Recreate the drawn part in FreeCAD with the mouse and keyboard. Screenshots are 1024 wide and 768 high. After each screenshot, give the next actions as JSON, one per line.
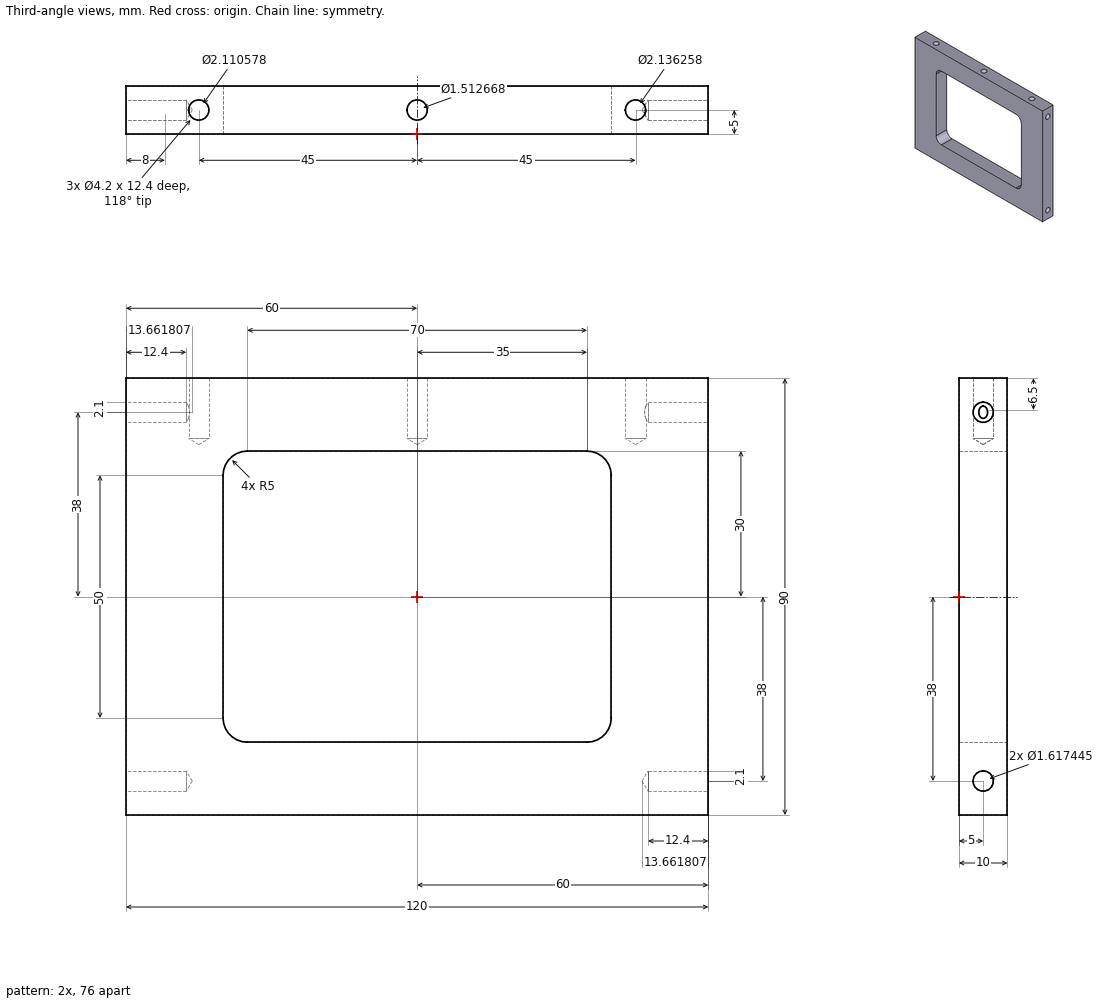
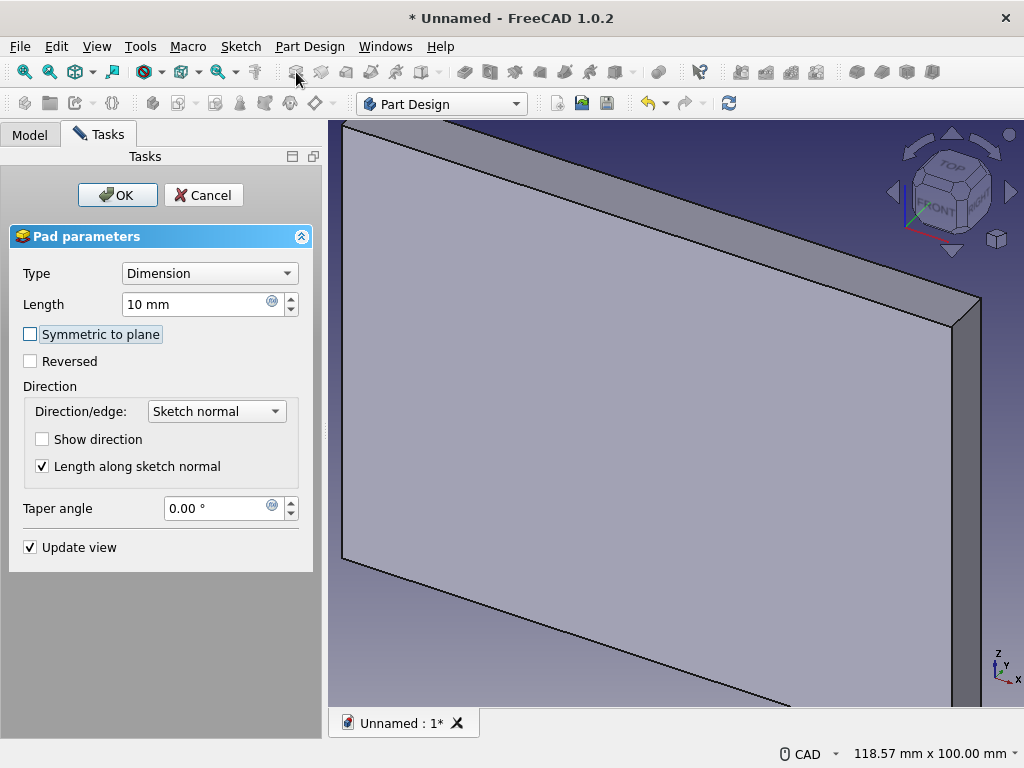
{"action": "left_click", "coordinate": [31, 361]}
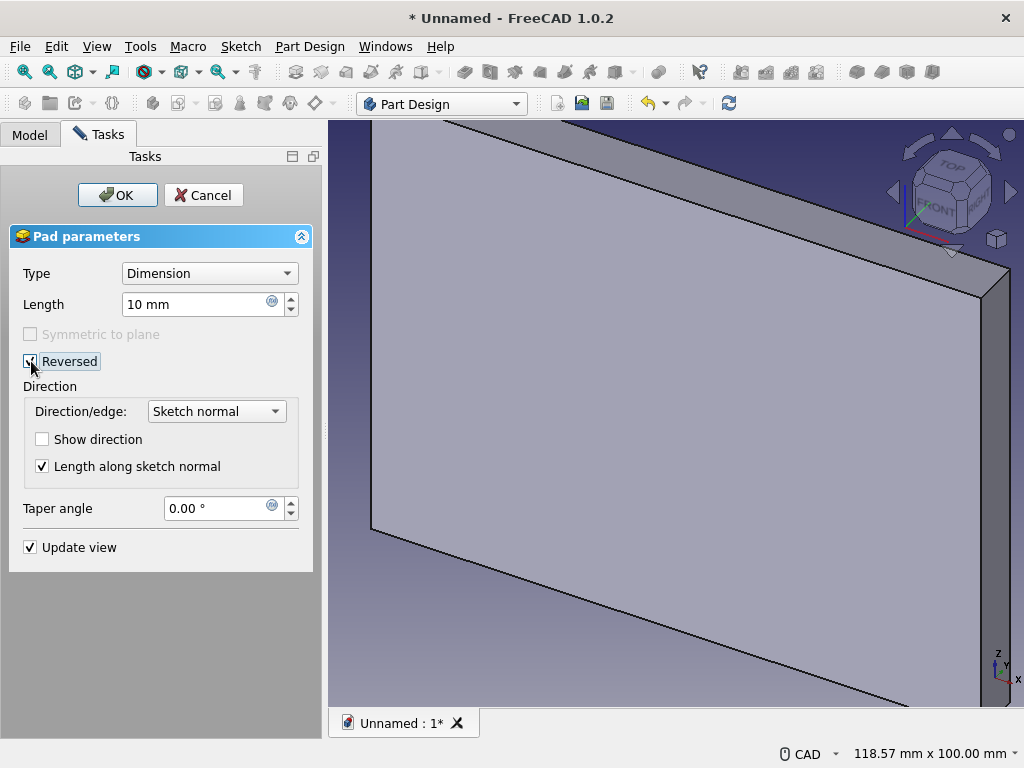
{"action": "left_click", "coordinate": [118, 195]}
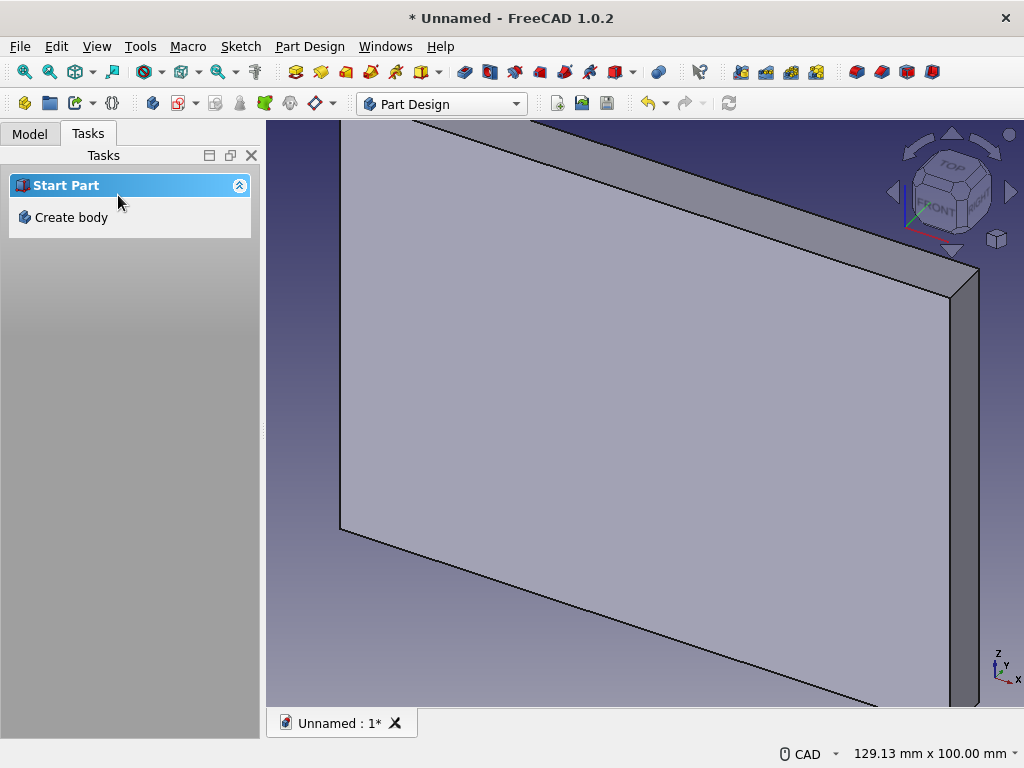
{"action": "left_click", "coordinate": [25, 72]}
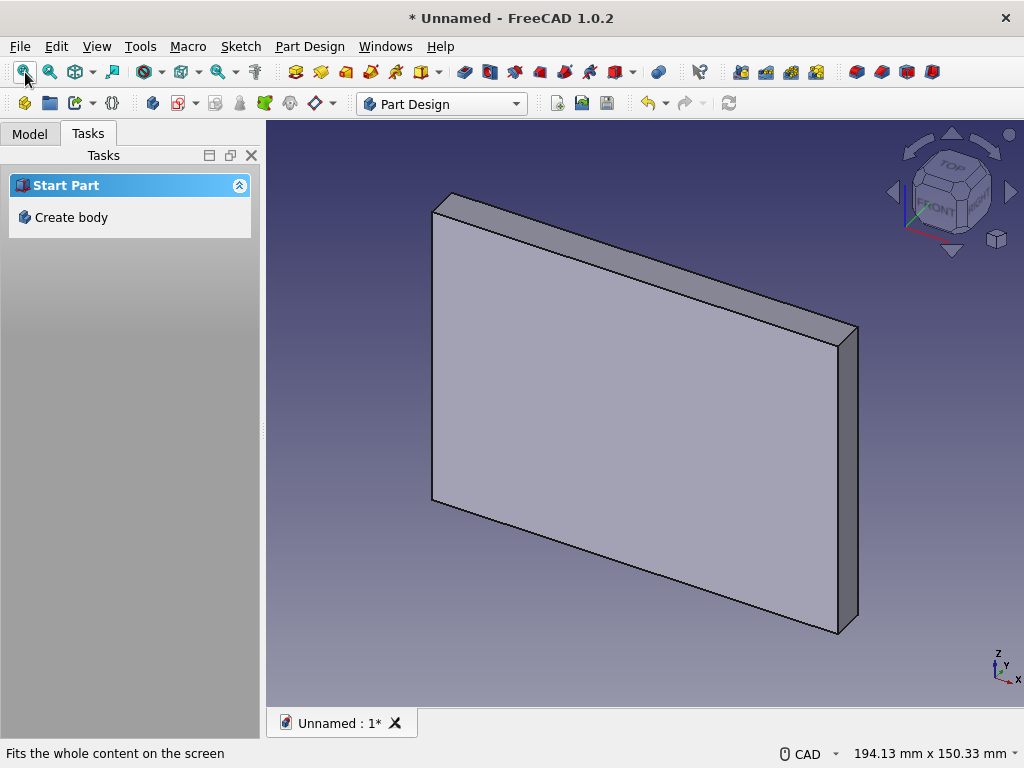
{"action": "key", "text": "6"}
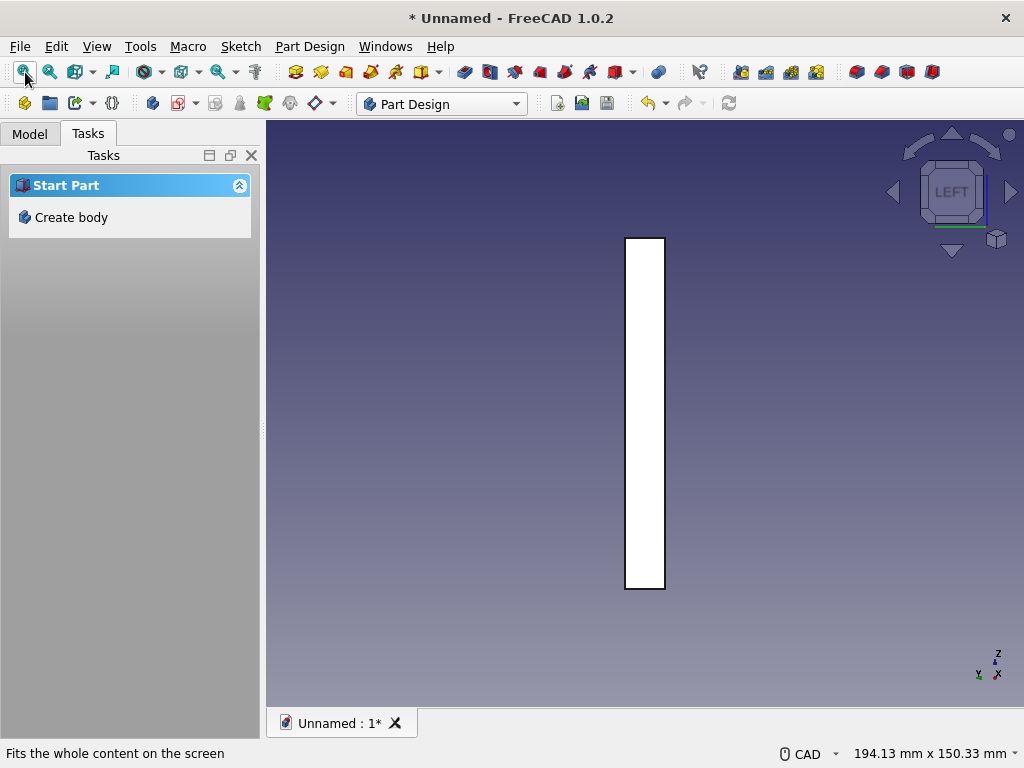
{"action": "left_click", "coordinate": [645, 262]}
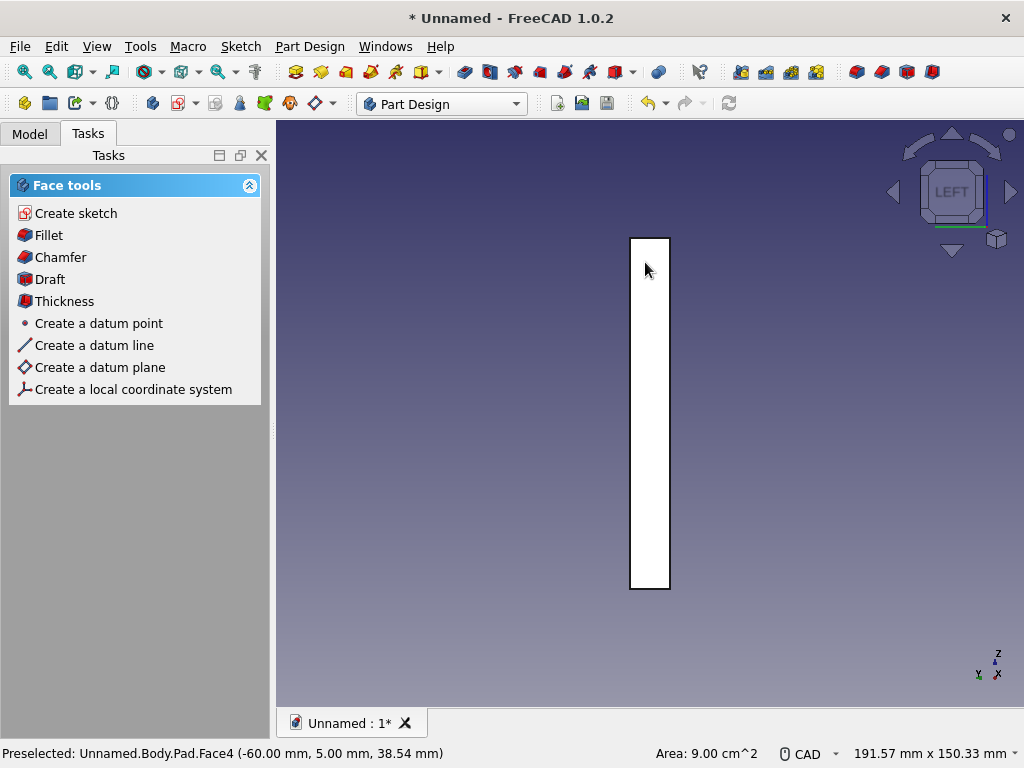
{"action": "left_click", "coordinate": [178, 104]}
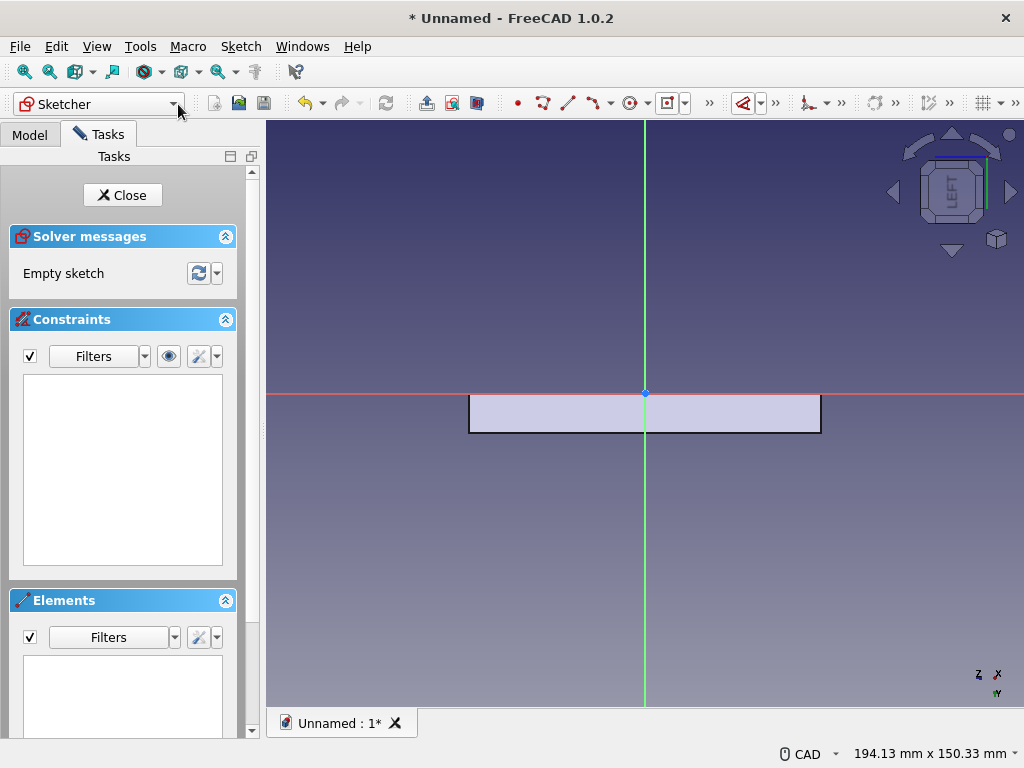
{"action": "left_click", "coordinate": [630, 104]}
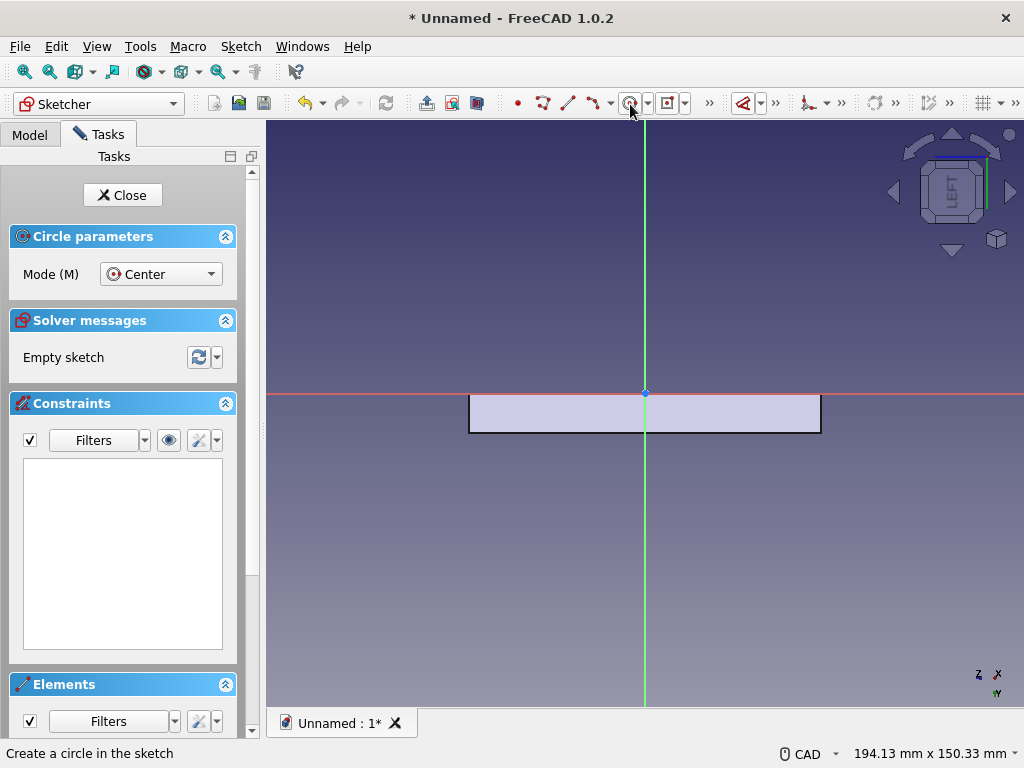
{"action": "scroll", "coordinate": [793, 414], "scroll_direction": "up", "scroll_amount": 10}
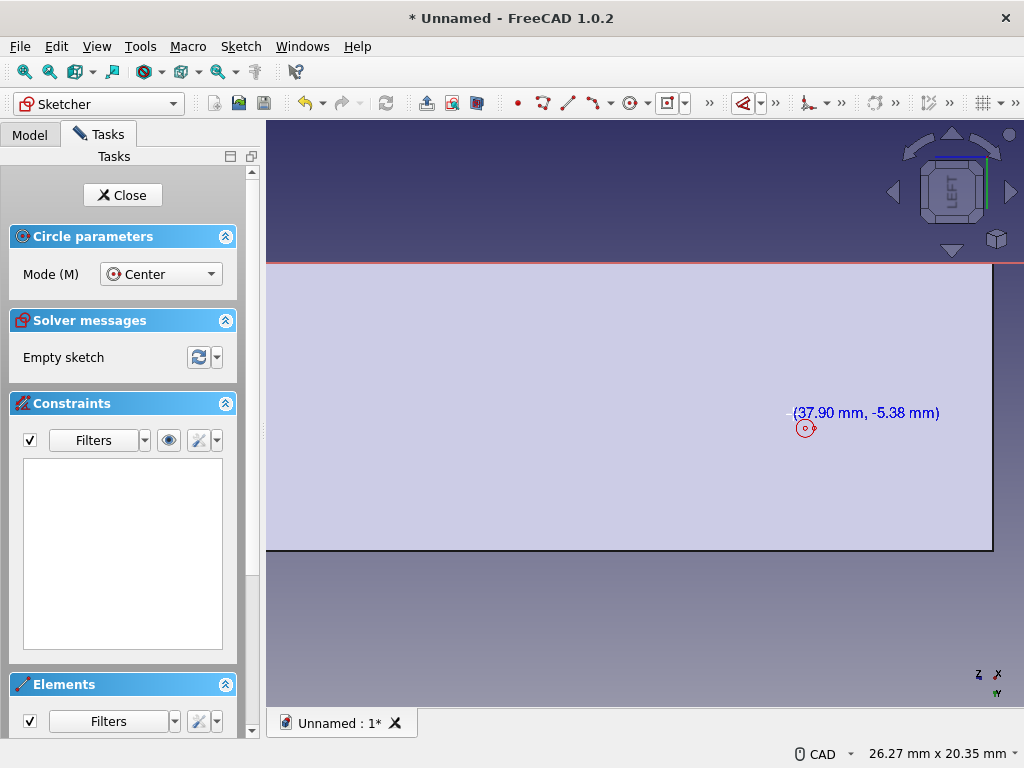
{"action": "scroll", "coordinate": [751, 427], "scroll_direction": "down", "scroll_amount": 9}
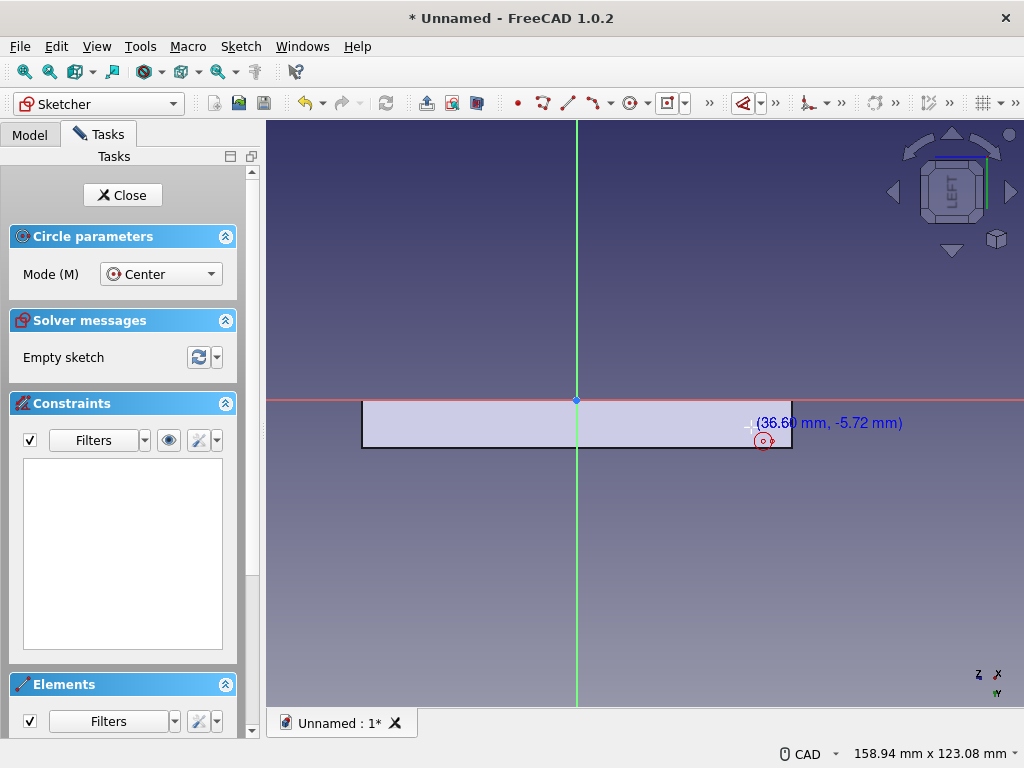
{"action": "left_click", "coordinate": [758, 424]}
{"action": "mouse_move", "coordinate": [761, 421]}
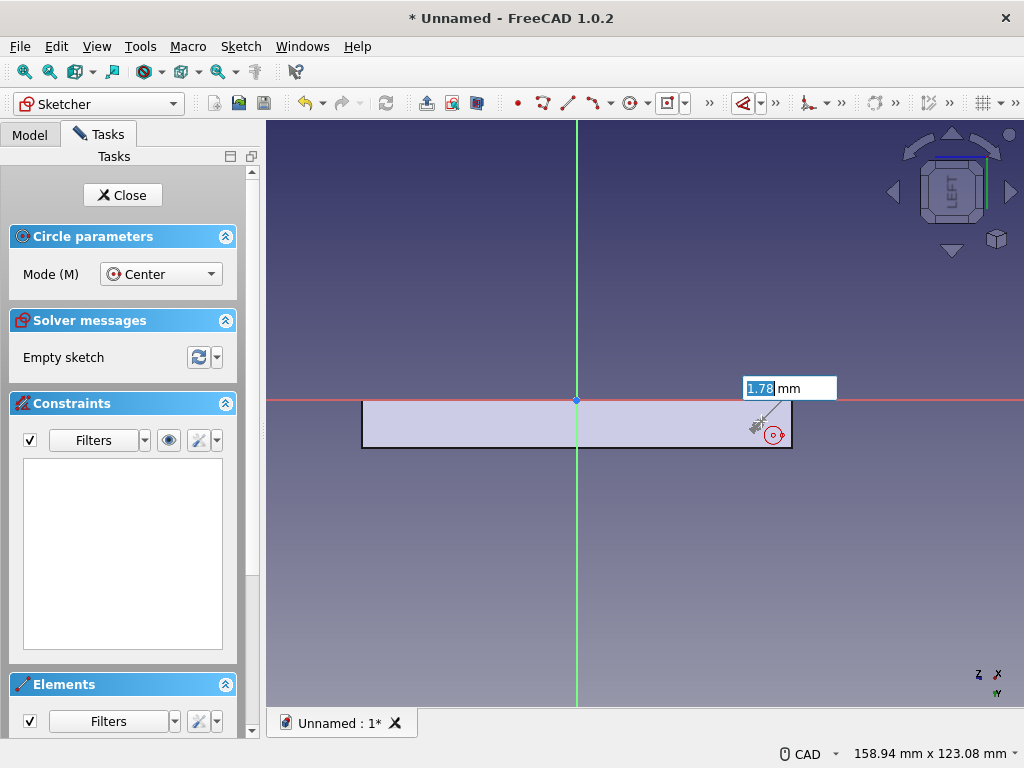
{"action": "type", "text": "1.617445"}
{"action": "key", "text": "Return"}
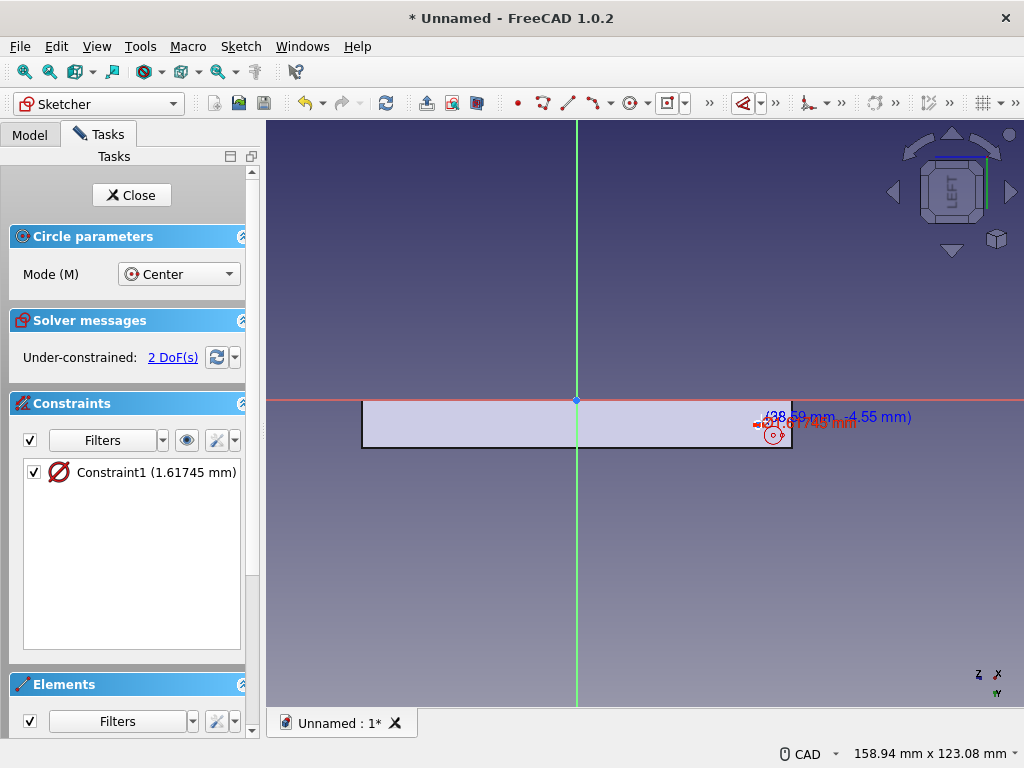
{"action": "scroll", "coordinate": [396, 424], "scroll_direction": "up", "scroll_amount": 9}